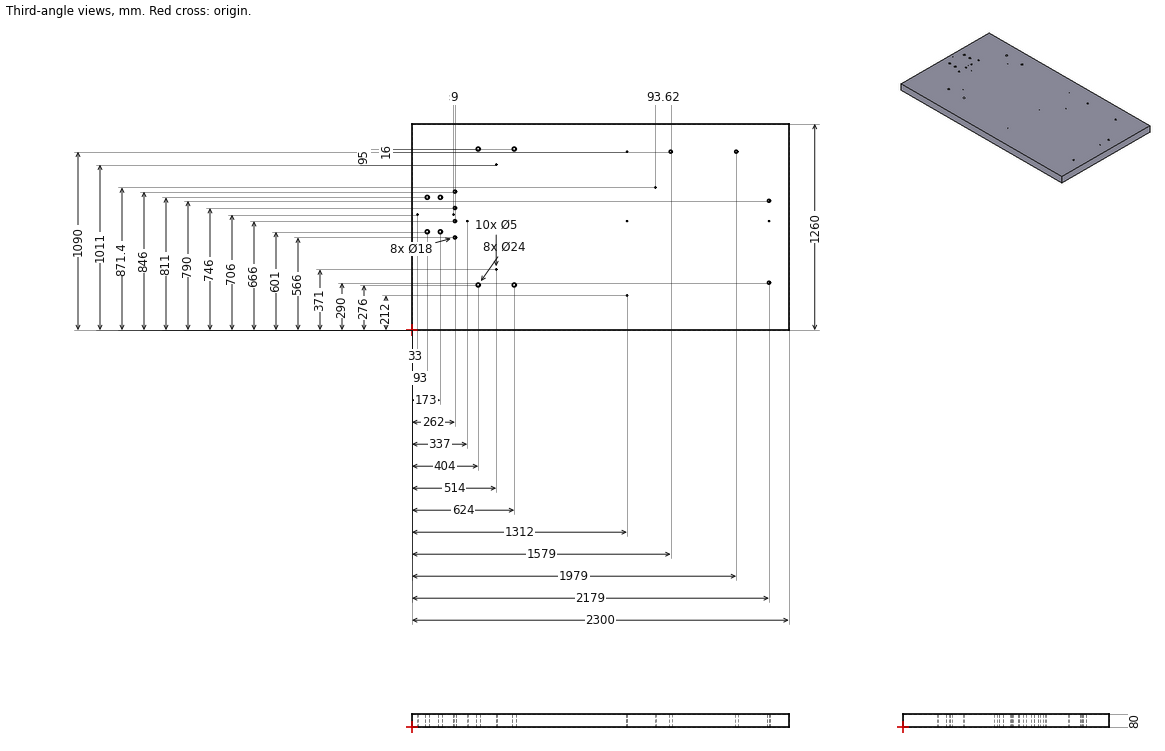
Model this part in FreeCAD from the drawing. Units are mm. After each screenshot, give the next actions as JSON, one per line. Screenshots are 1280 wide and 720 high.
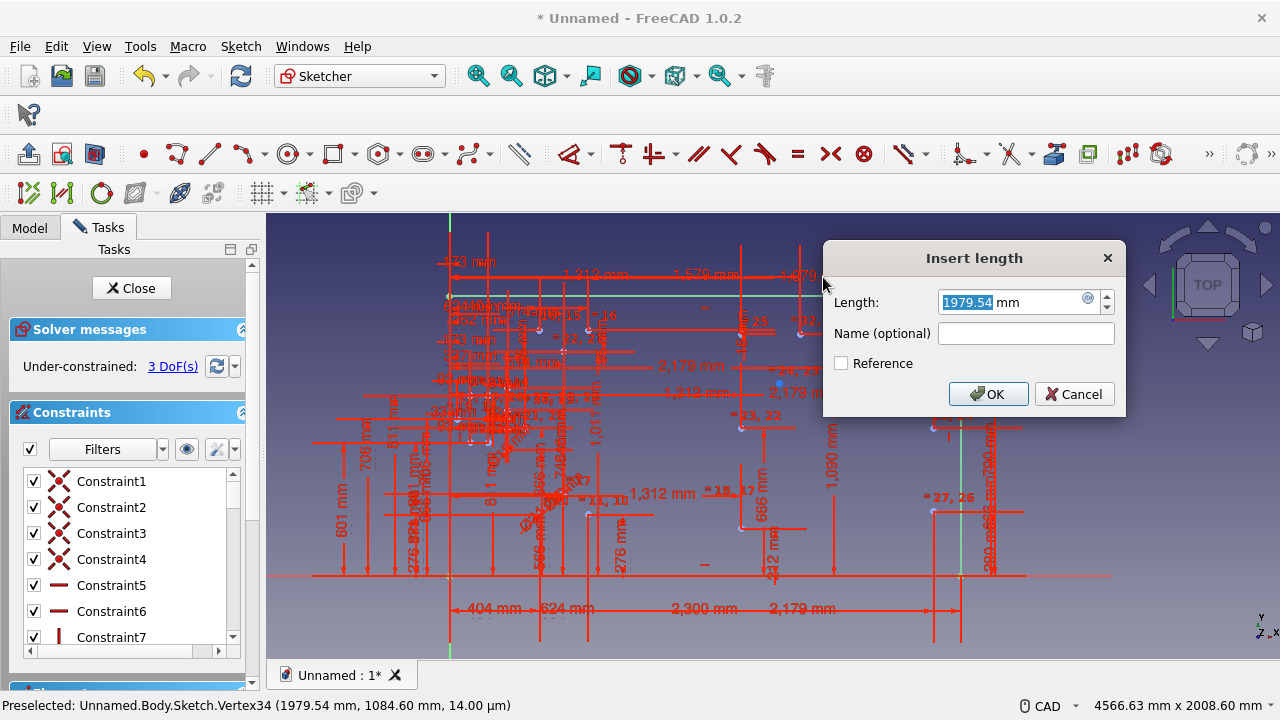
{"action": "type", "text": "1979"}
{"action": "key", "text": "Return"}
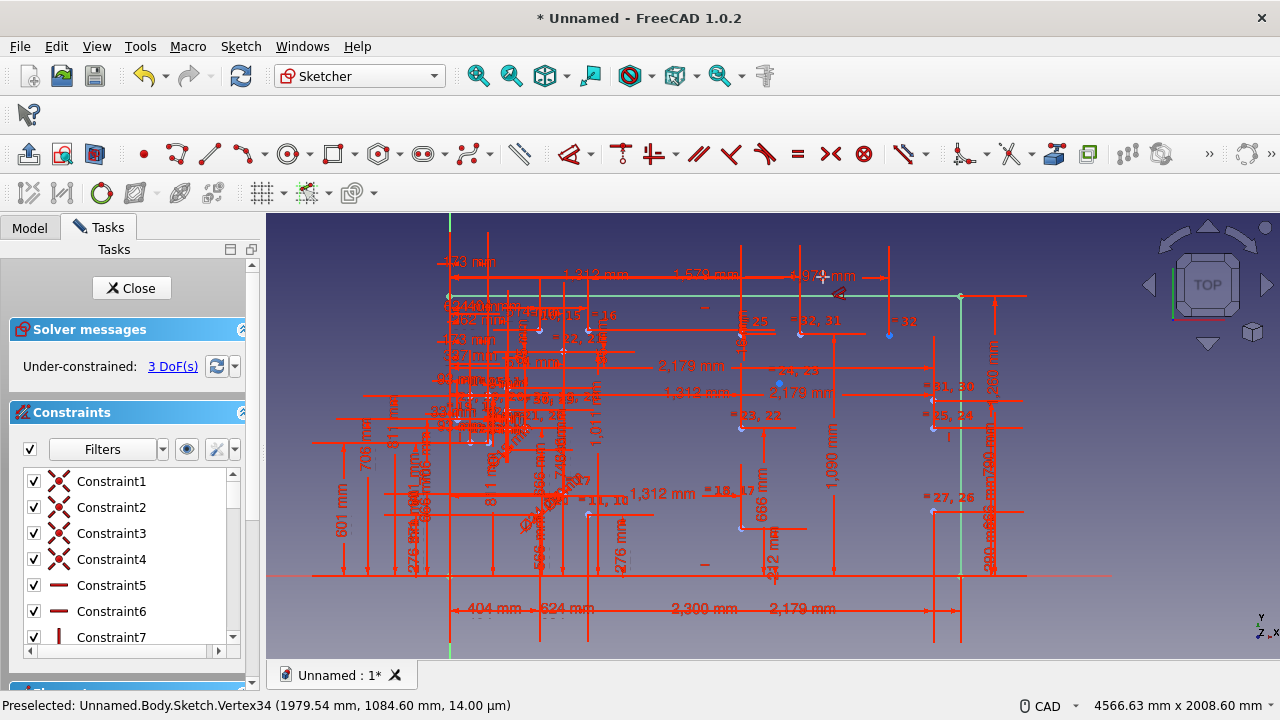
{"action": "left_click", "coordinate": [889, 335]}
{"action": "left_click", "coordinate": [923, 371]}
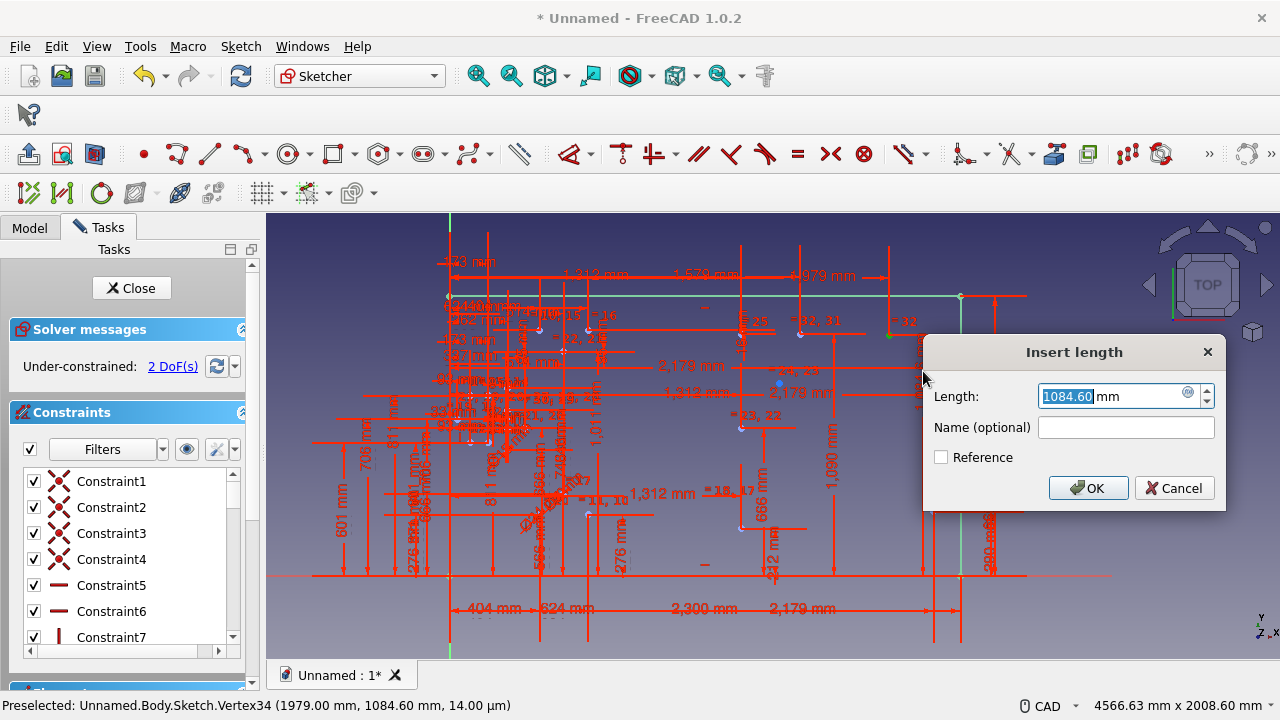
{"action": "type", "text": "1090"}
{"action": "key", "text": "Return"}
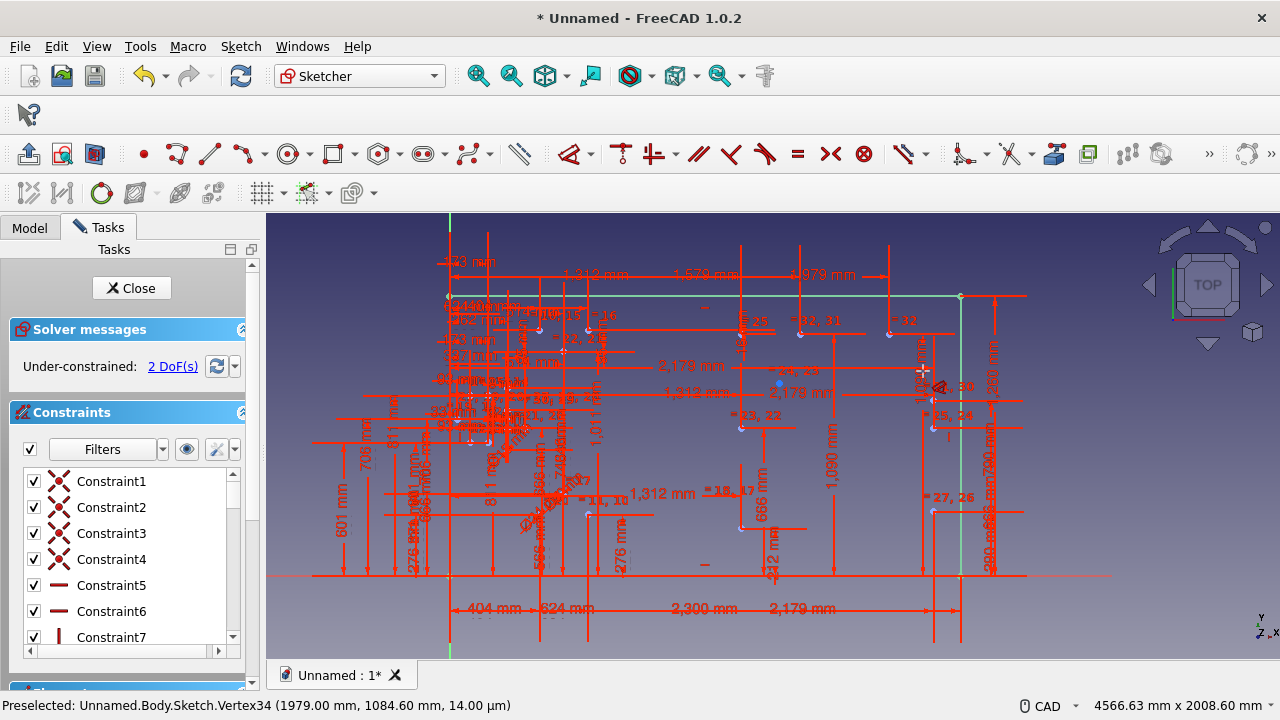
{"action": "left_click", "coordinate": [779, 384]}
{"action": "left_click", "coordinate": [813, 524]}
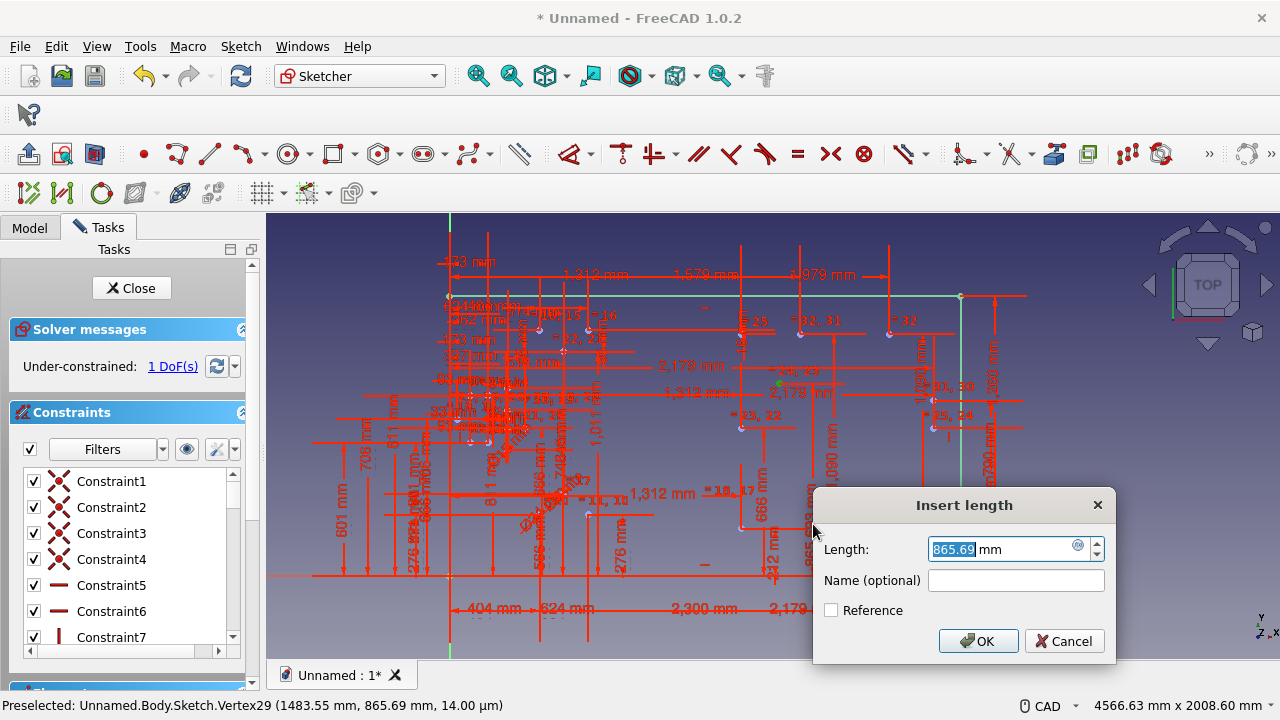
{"action": "type", "text": "871.4"}
{"action": "key", "text": "Return"}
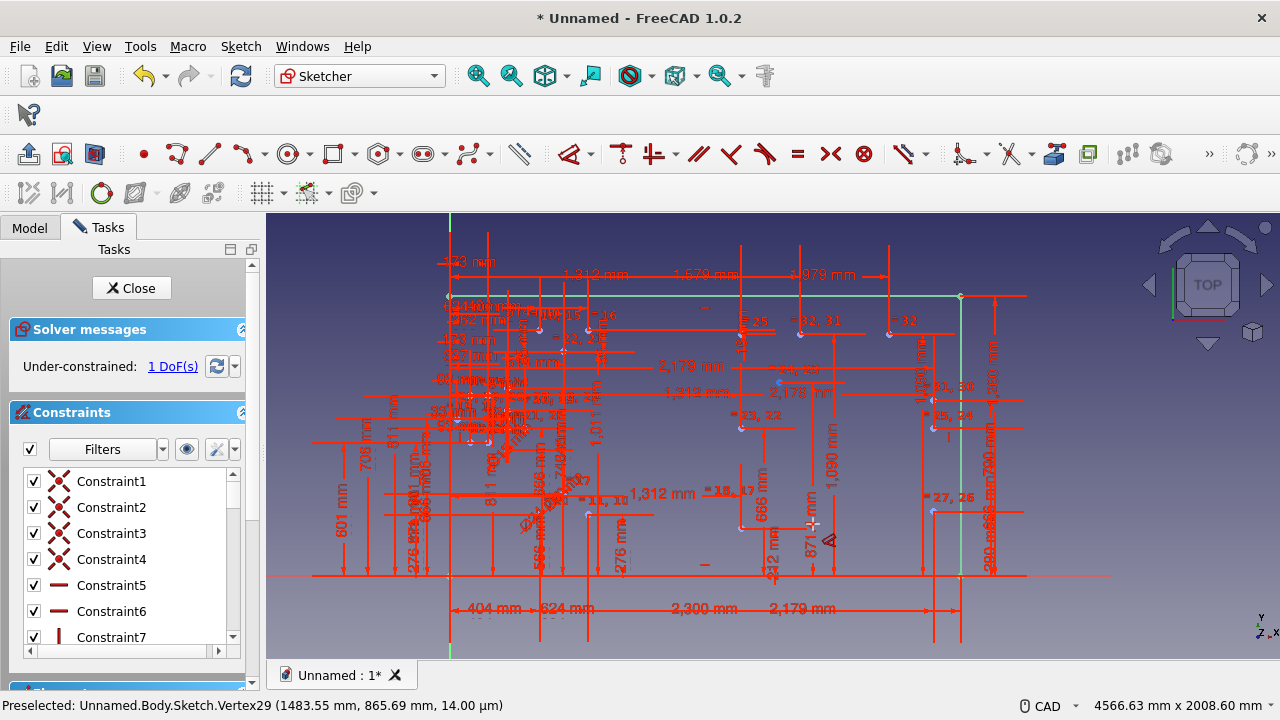
{"action": "scroll", "coordinate": [779, 383], "scroll_direction": "up", "scroll_amount": 4}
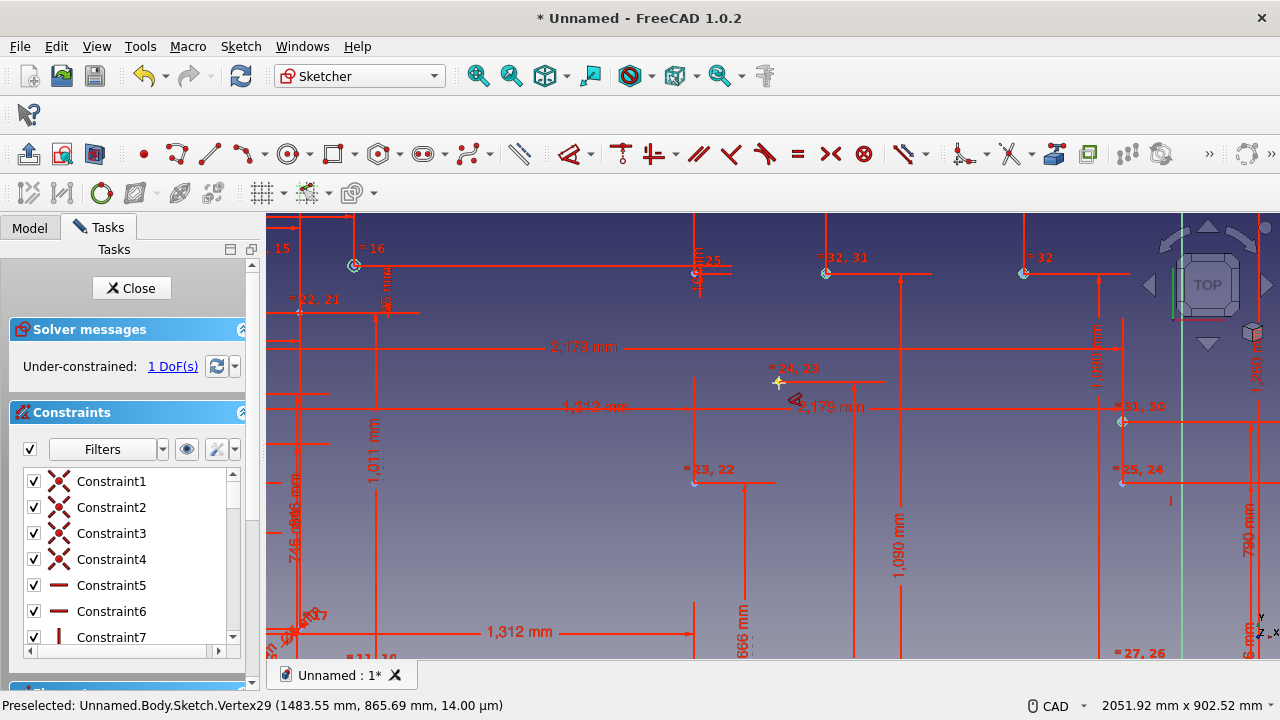
{"action": "left_click", "coordinate": [779, 382]}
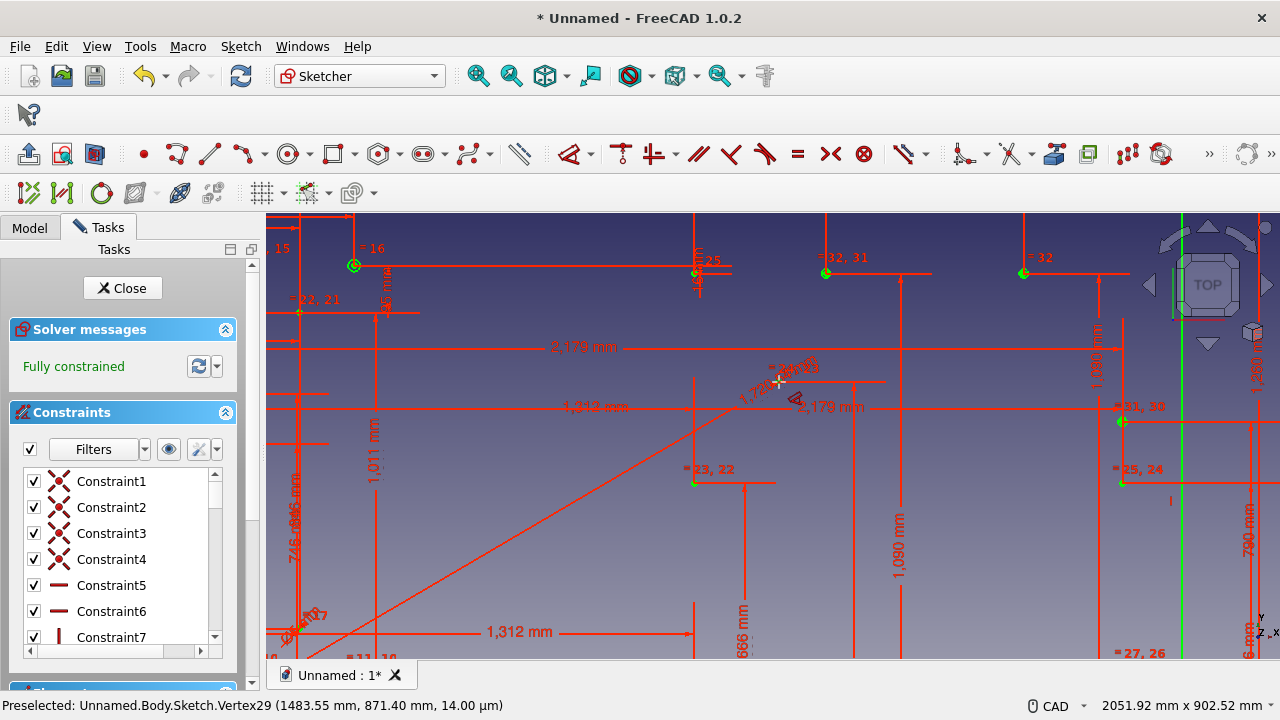
{"action": "left_click", "coordinate": [826, 274]}
{"action": "left_click", "coordinate": [802, 440]}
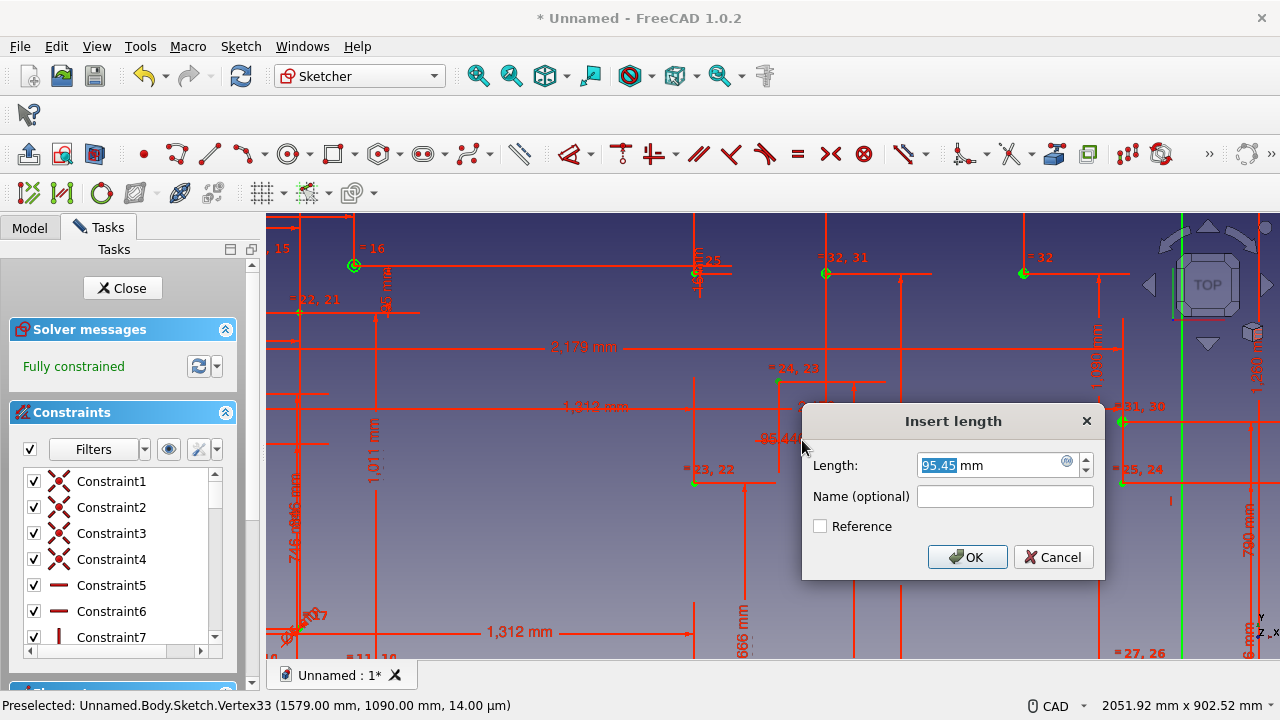
{"action": "type", "text": "93.62"}
{"action": "key", "text": "Return"}
{"action": "key", "text": "Escape"}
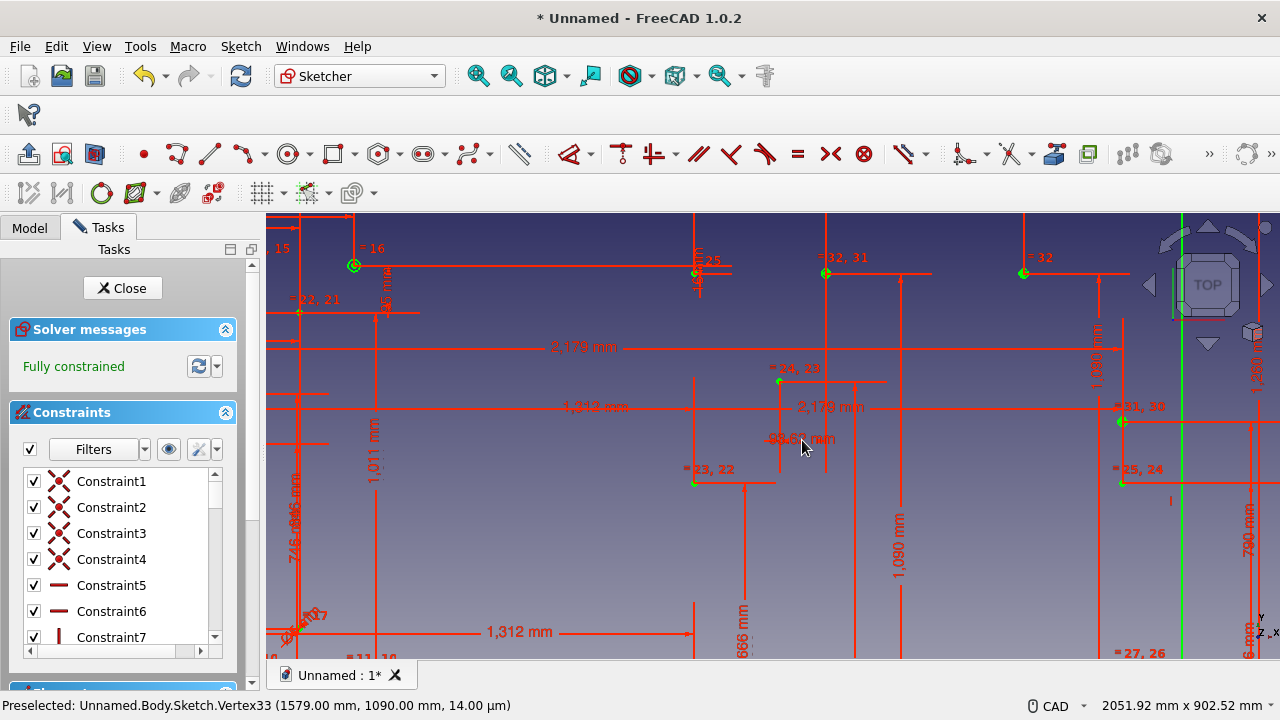
{"action": "left_click", "coordinate": [123, 288]}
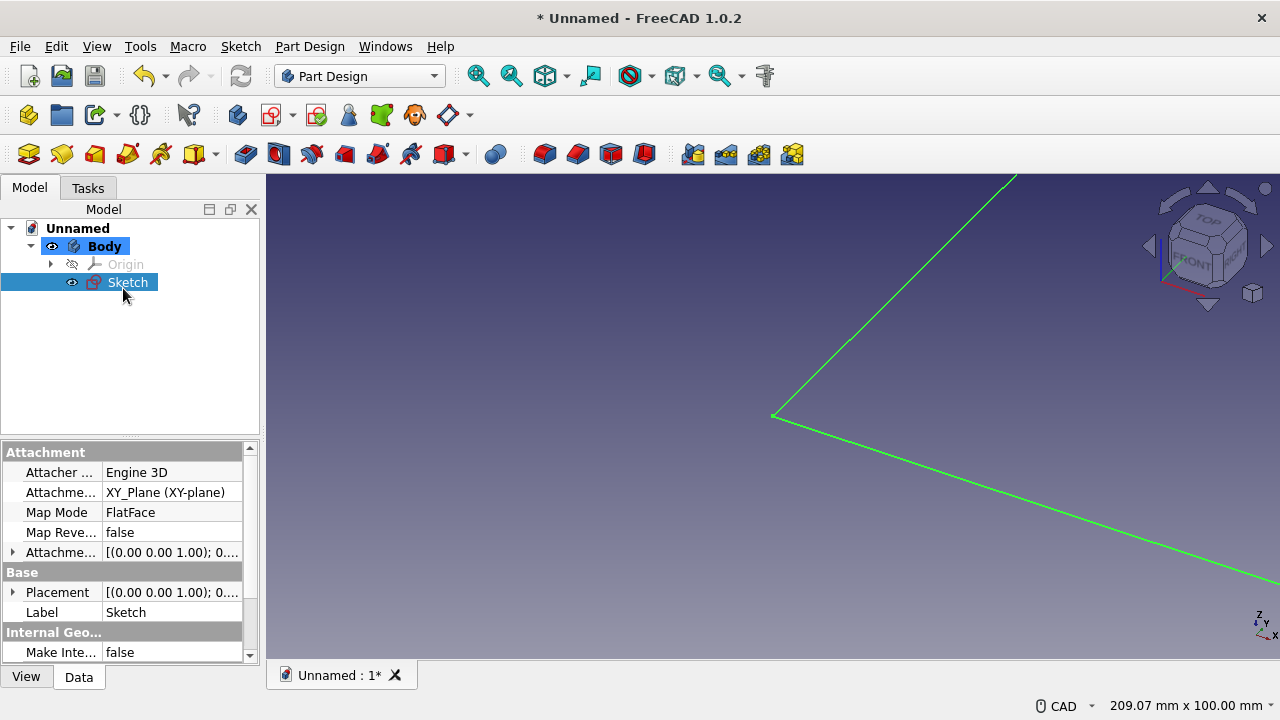
{"action": "left_click", "coordinate": [29, 154]}